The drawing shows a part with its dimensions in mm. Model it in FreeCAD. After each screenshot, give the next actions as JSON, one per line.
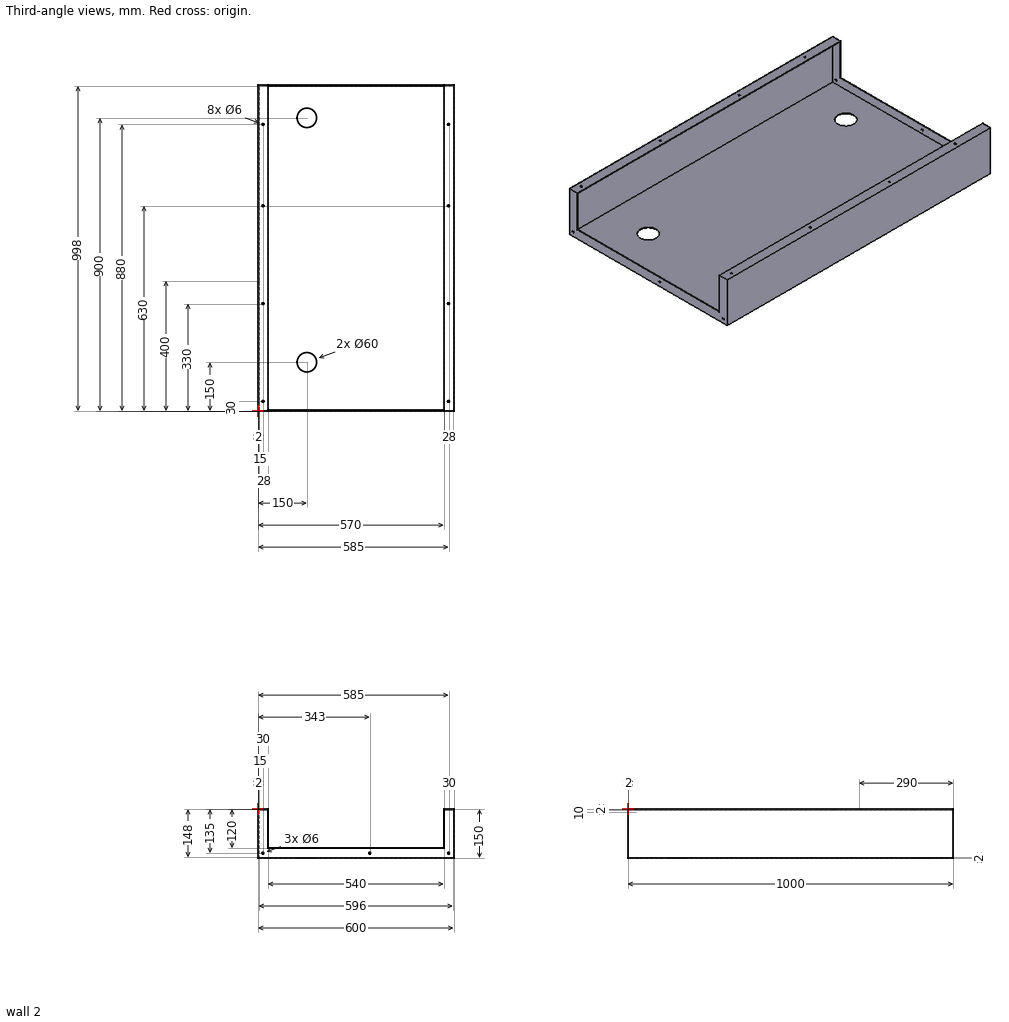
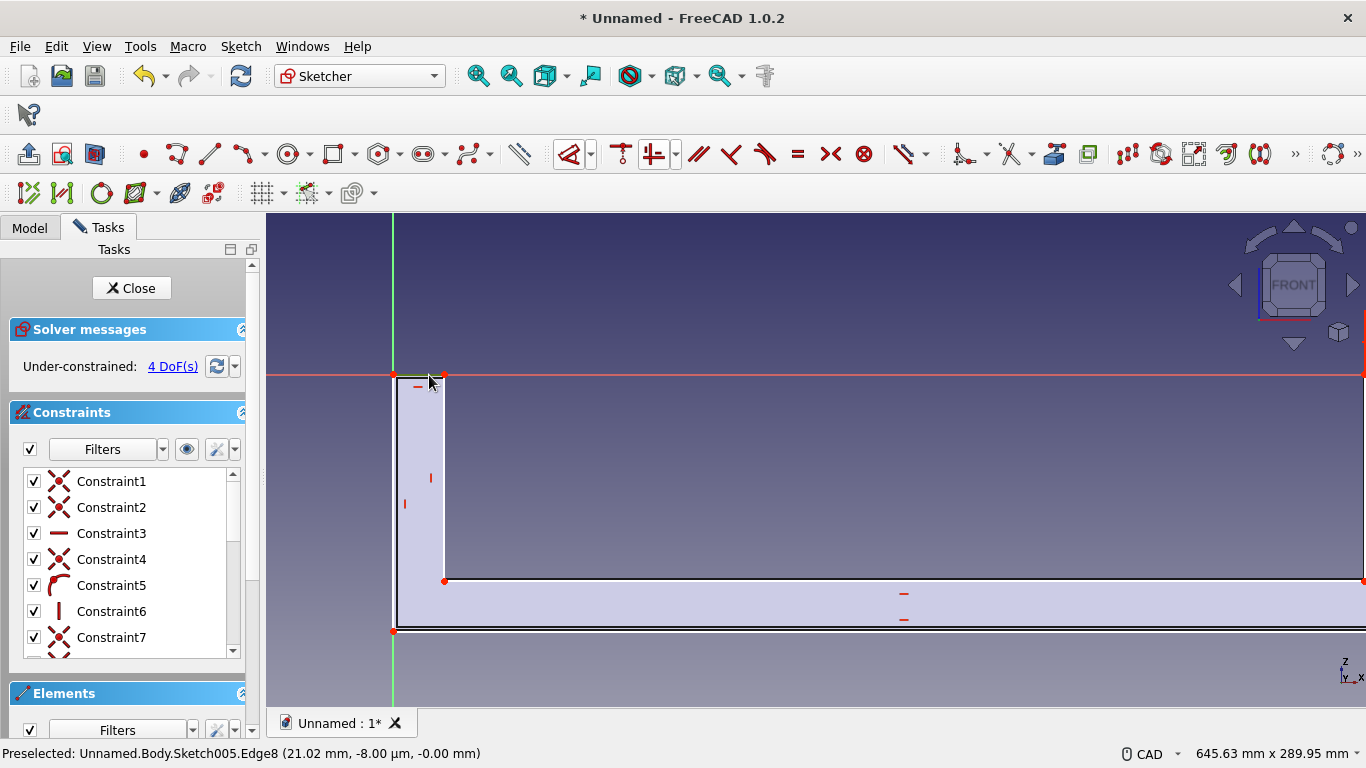
{"action": "left_click", "coordinate": [590, 154]}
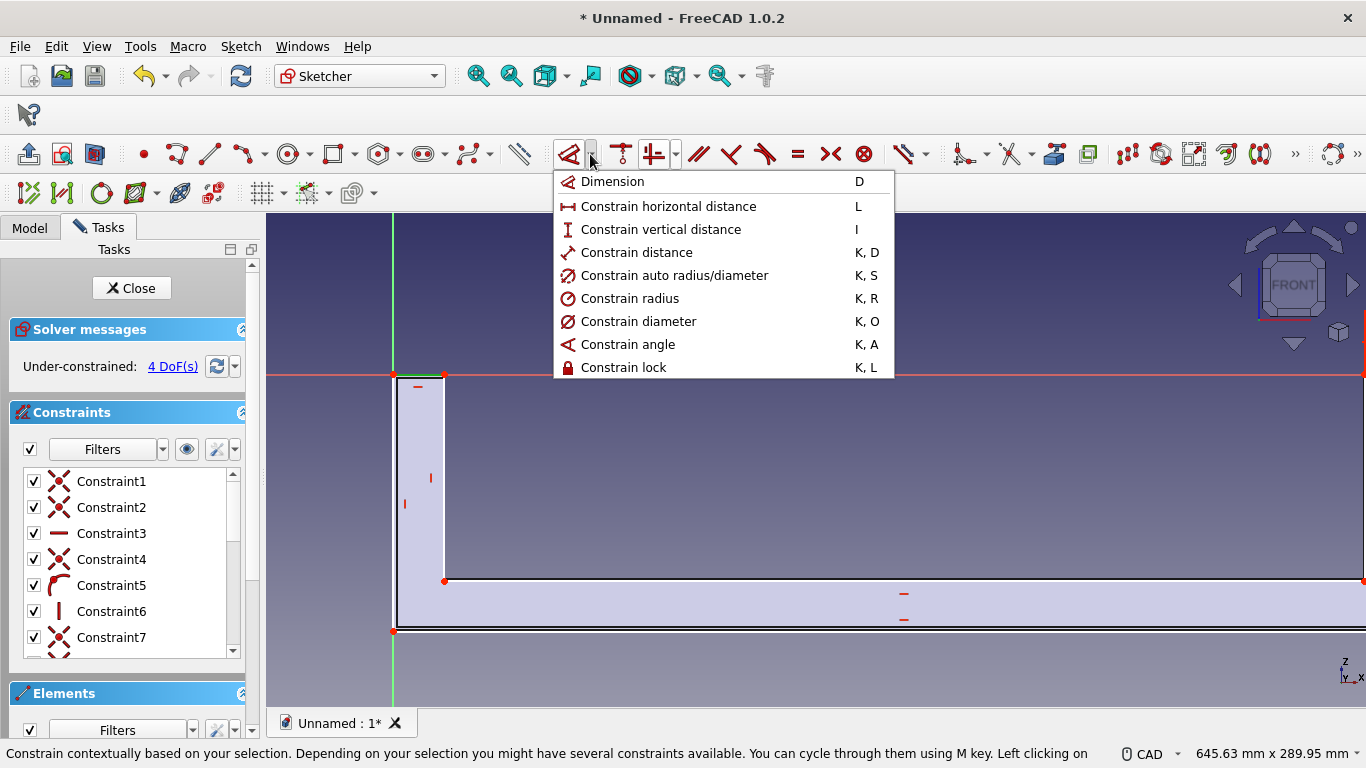
{"action": "left_click", "coordinate": [724, 206]}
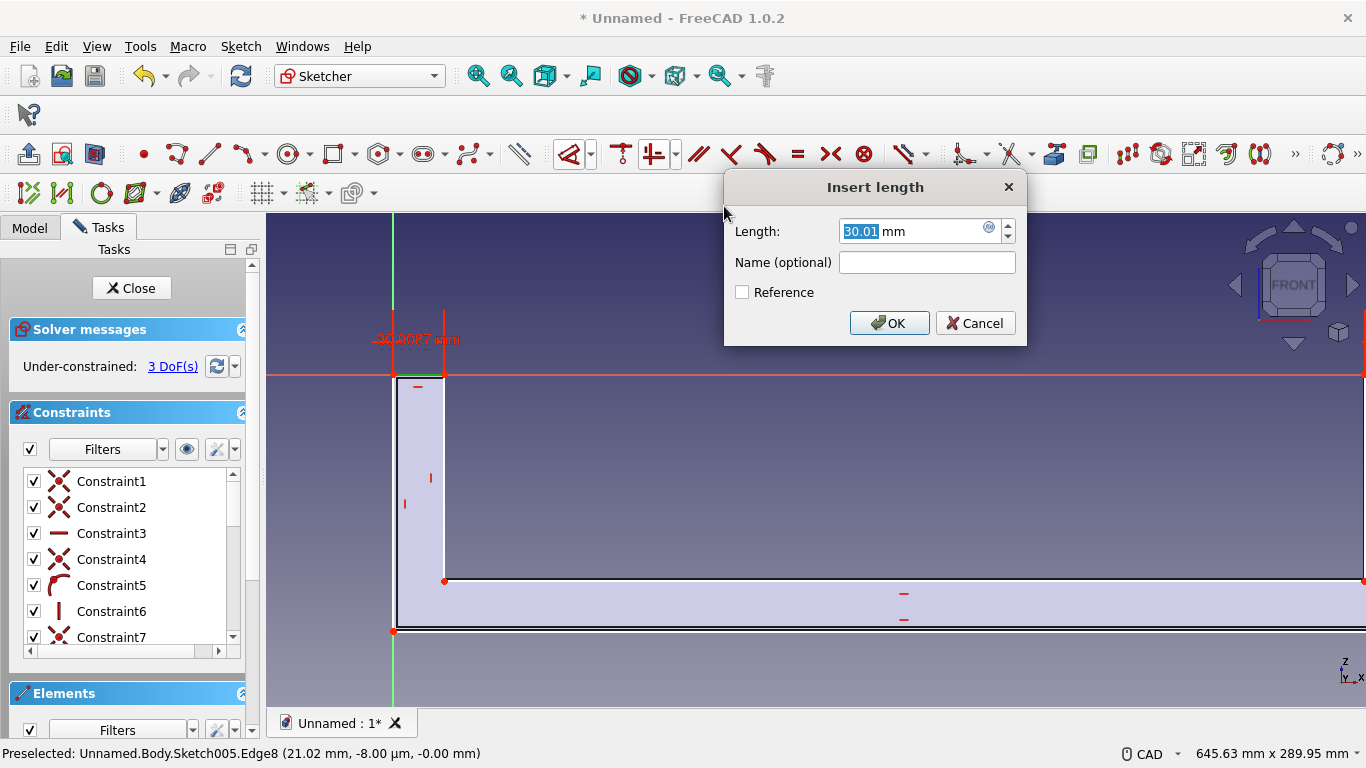
{"action": "type", "text": "30"}
{"action": "key", "text": "Return"}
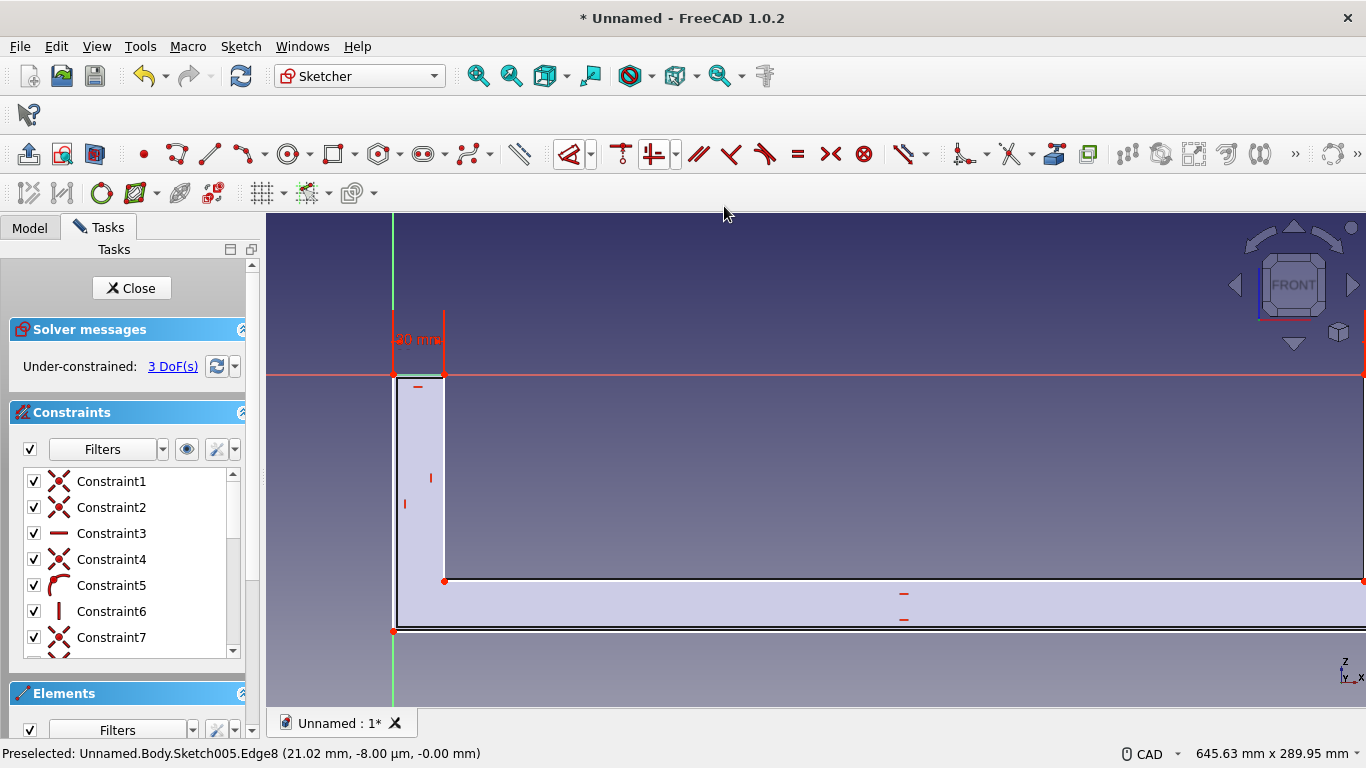
{"action": "left_click", "coordinate": [393, 452]}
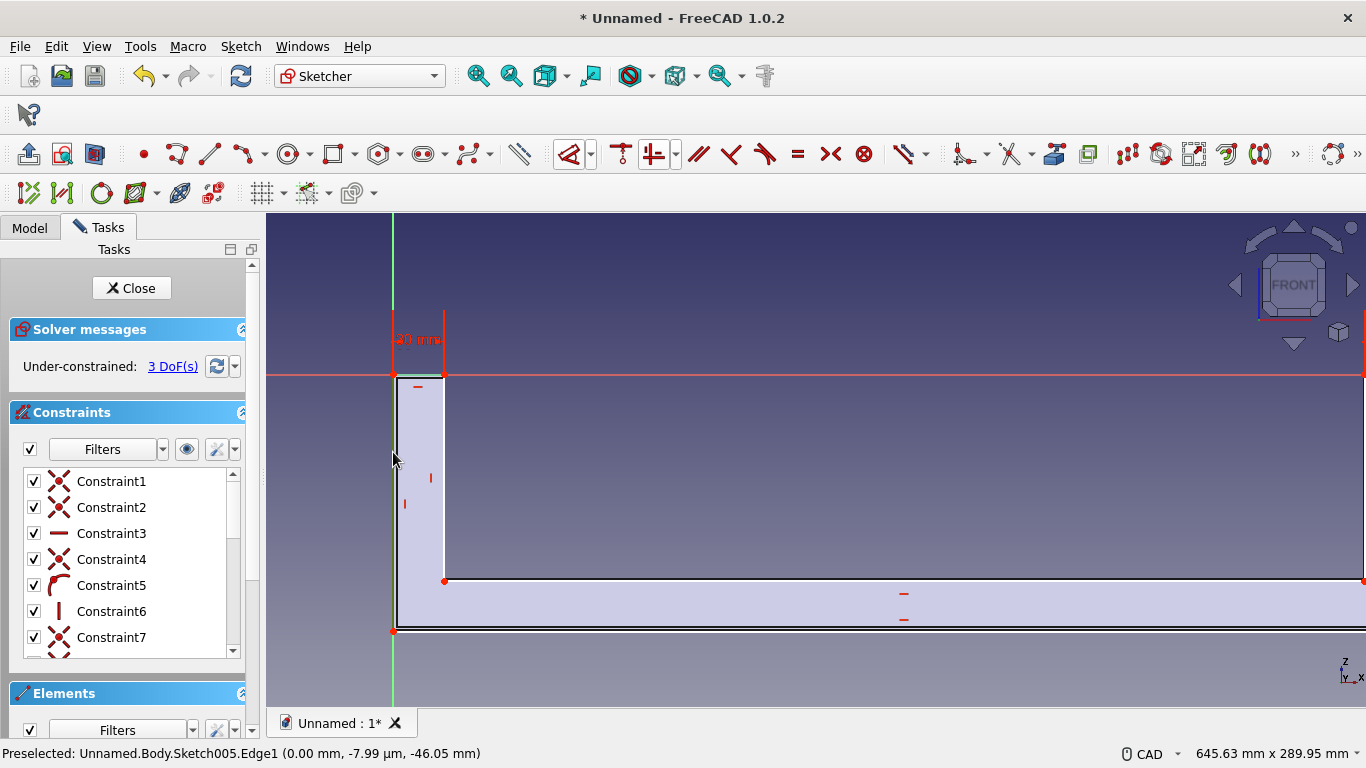
{"action": "left_click", "coordinate": [590, 154]}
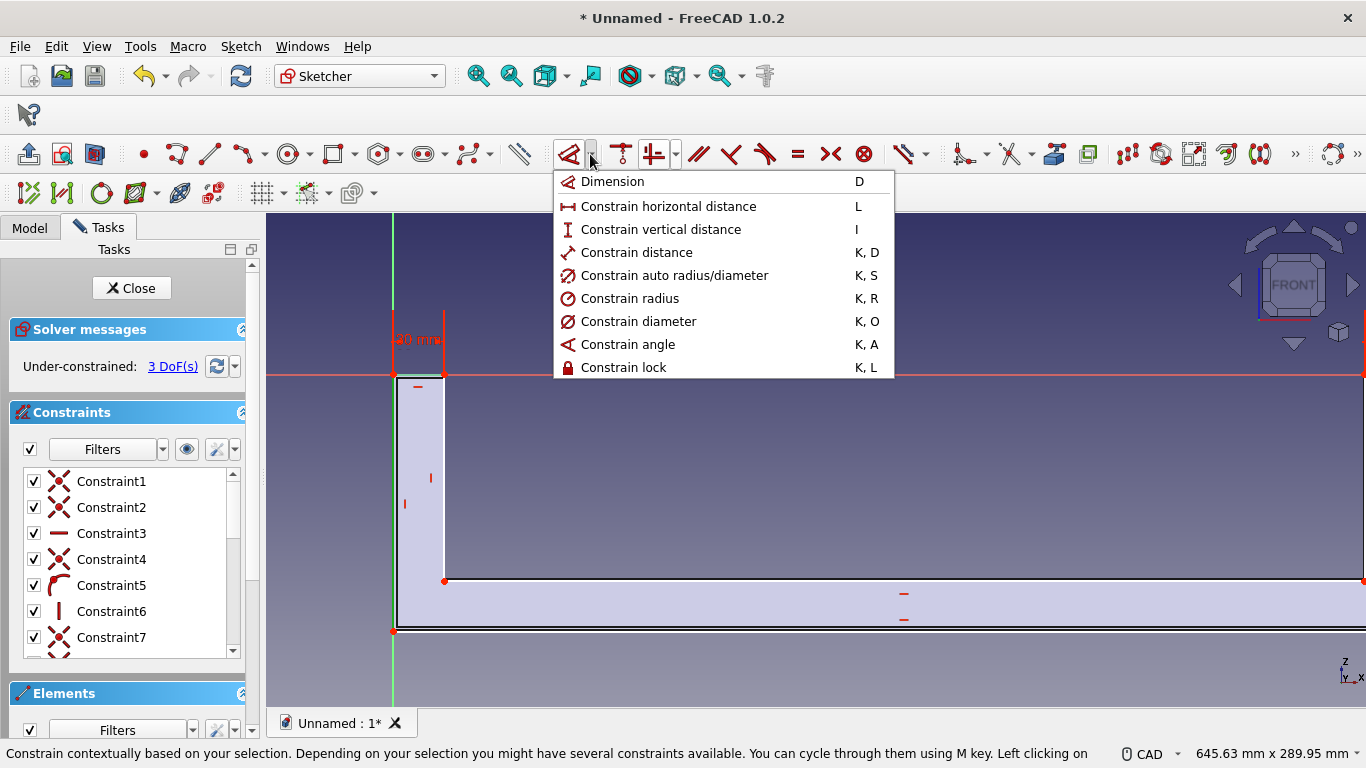
{"action": "left_click", "coordinate": [724, 230]}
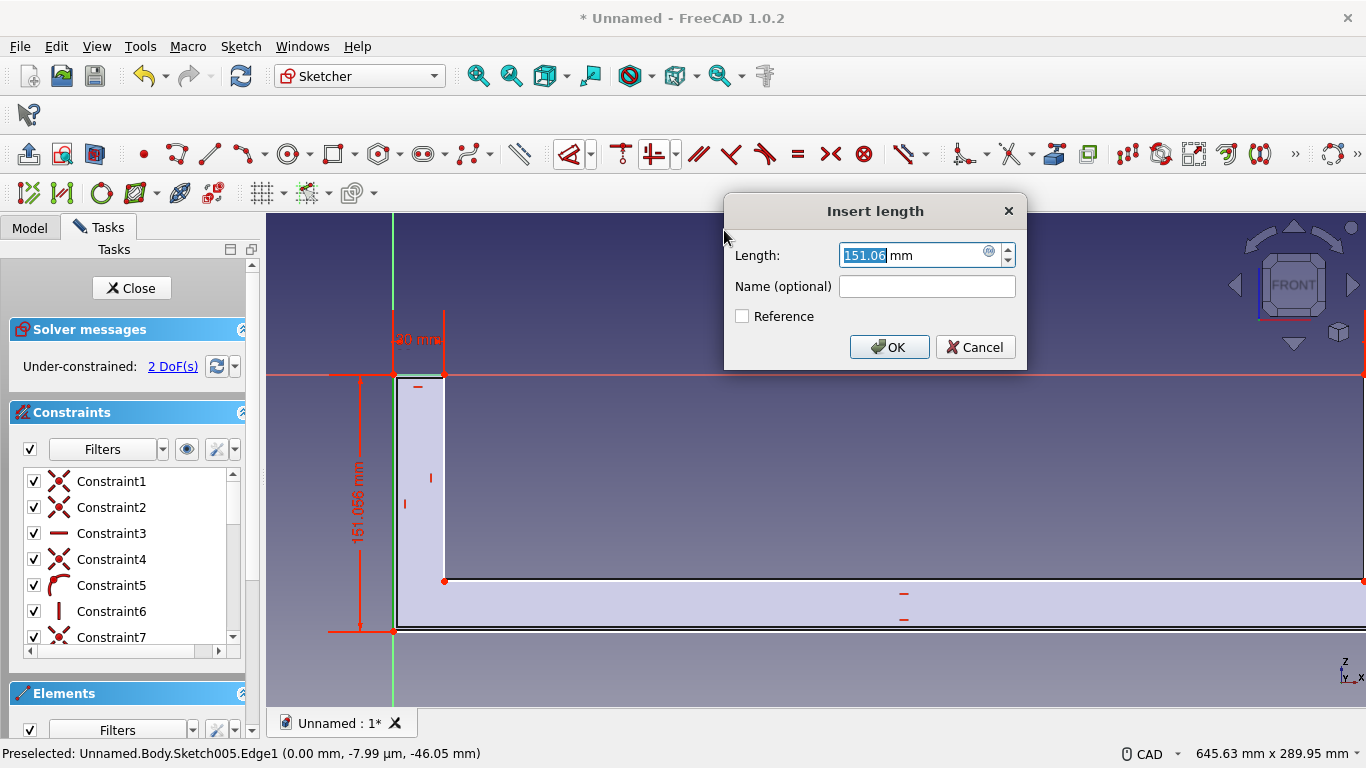
{"action": "type", "text": "150"}
{"action": "key", "text": "Return"}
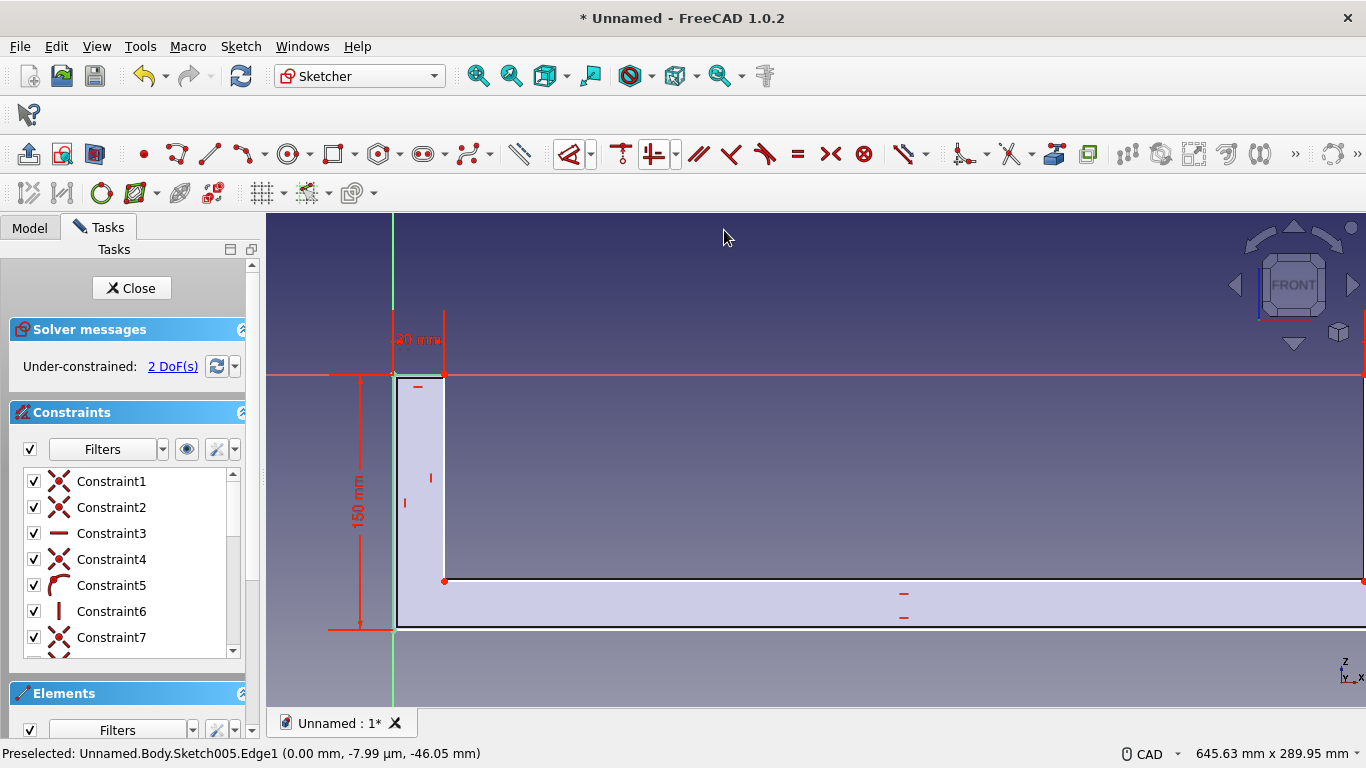
{"action": "left_click", "coordinate": [700, 630]}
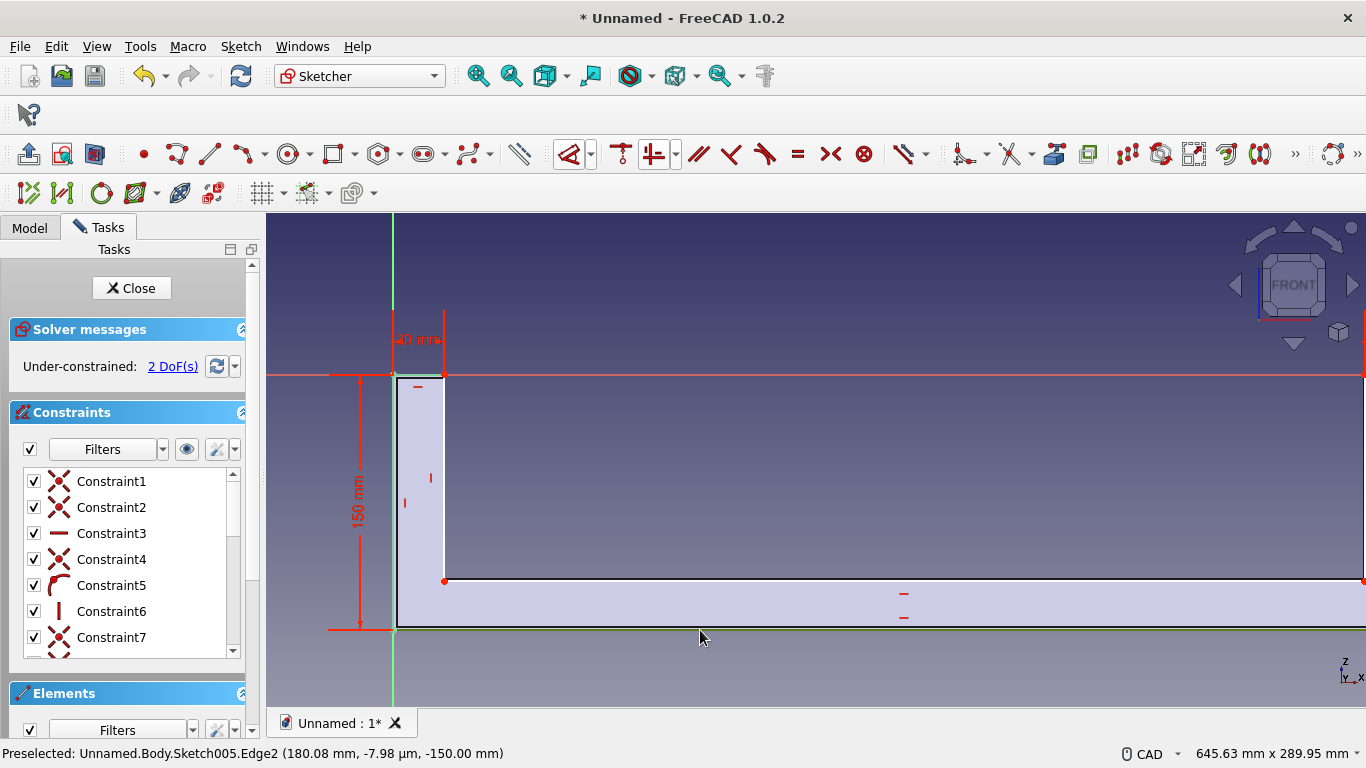
{"action": "left_click", "coordinate": [590, 154]}